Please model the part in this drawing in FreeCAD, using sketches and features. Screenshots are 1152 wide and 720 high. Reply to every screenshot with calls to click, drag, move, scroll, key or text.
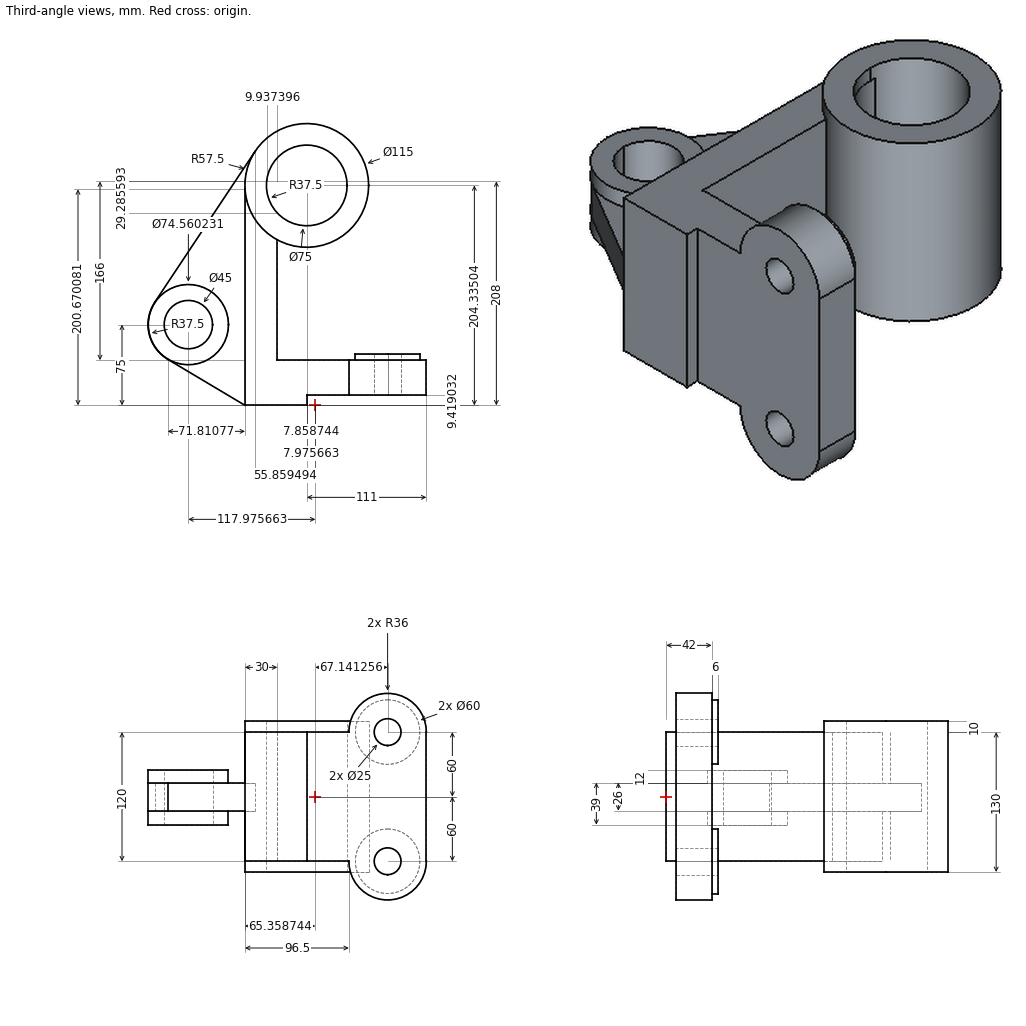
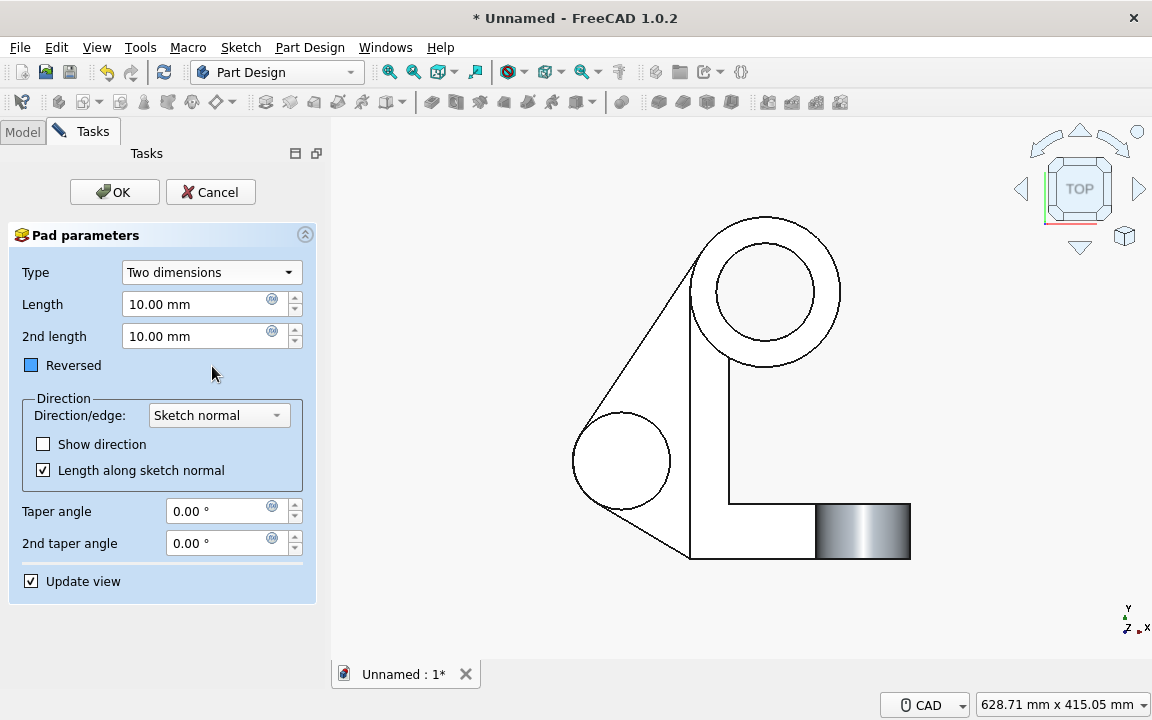
triple_click(204, 304)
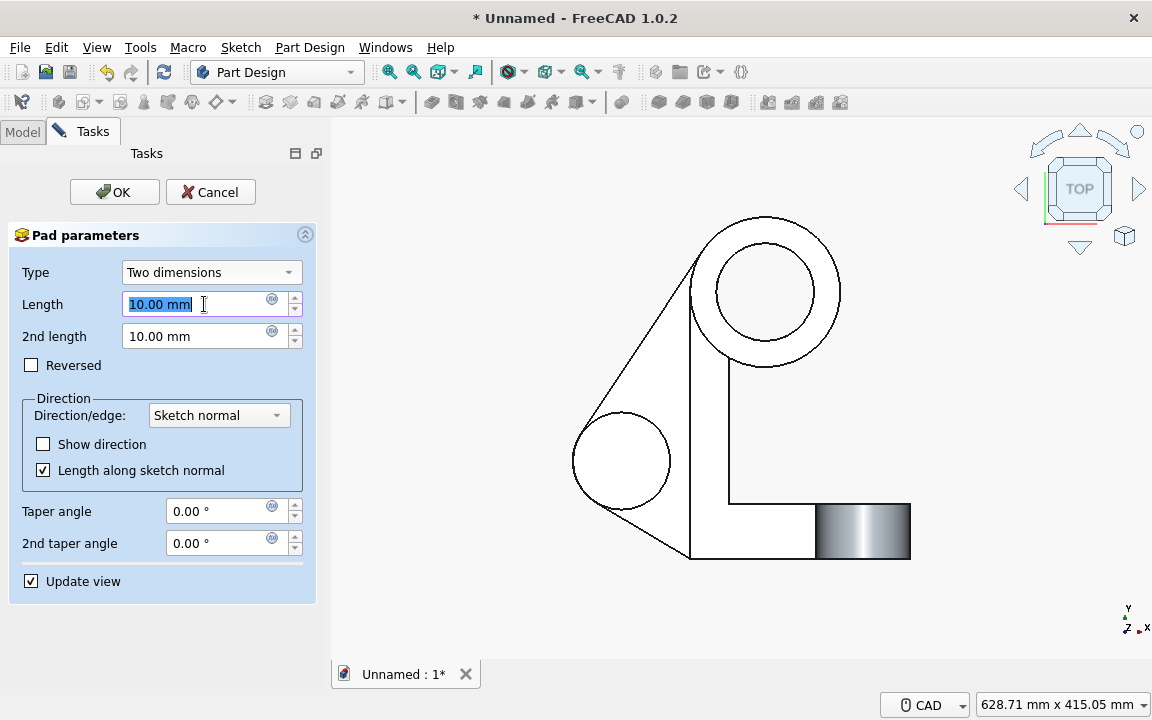
text(12)
key(Tab)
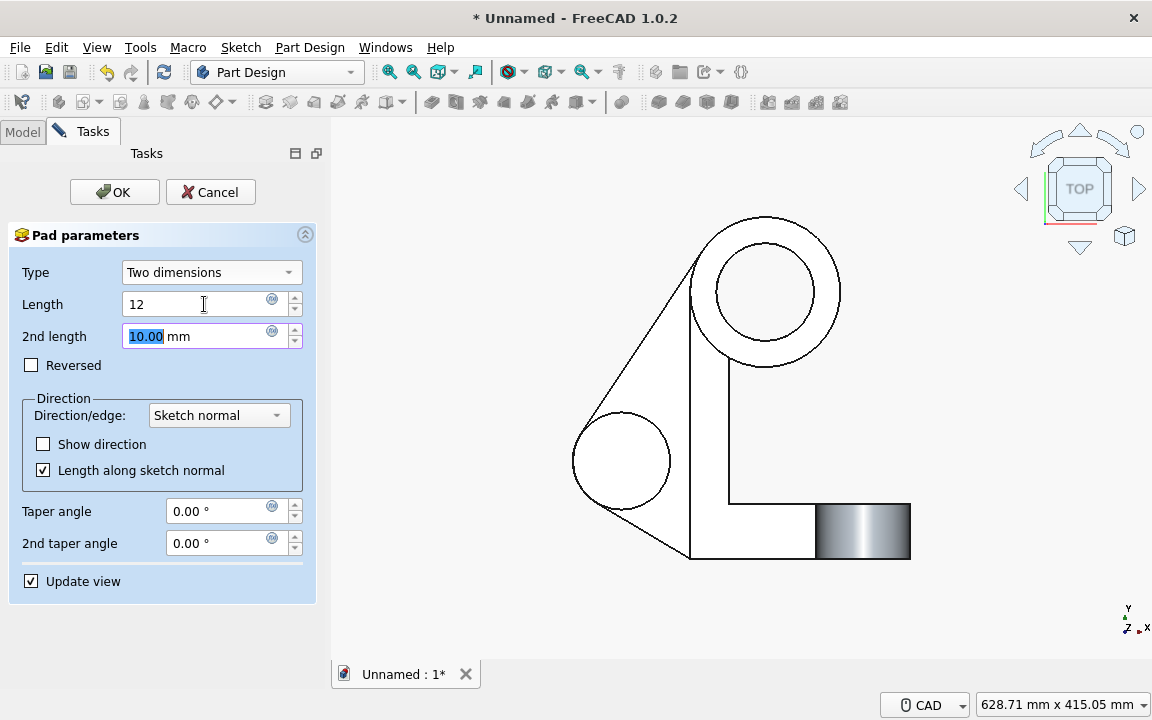
text(39)
key(Tab)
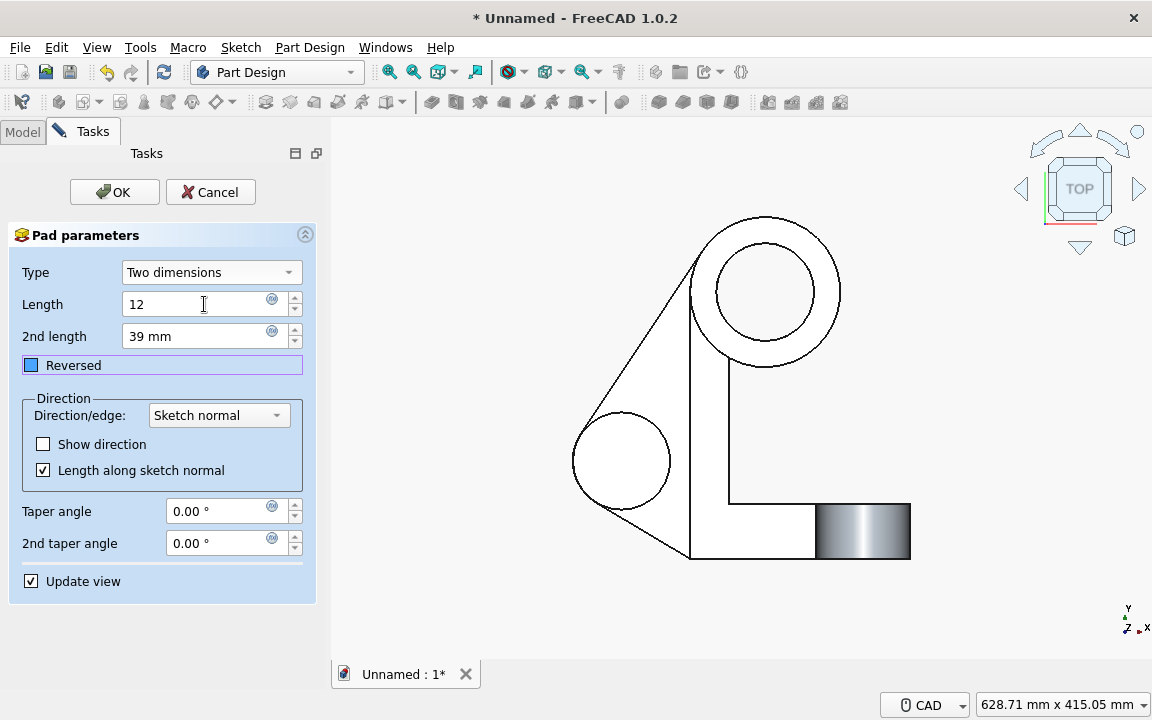
click(115, 192)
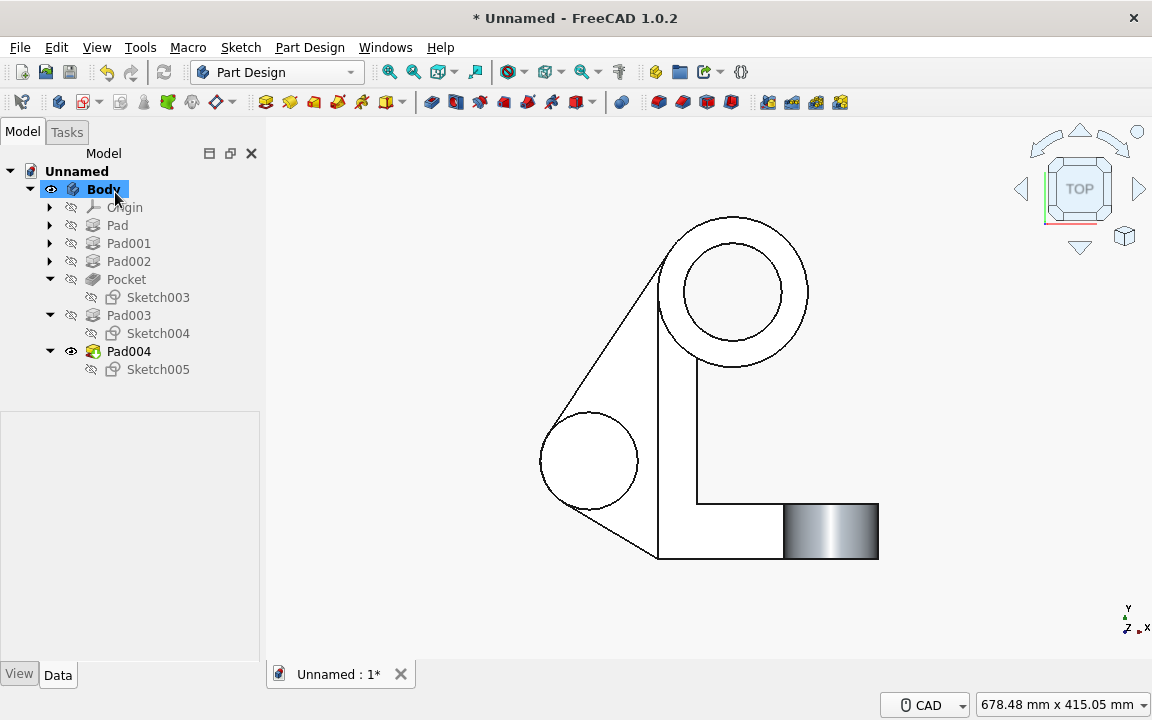
click(589, 460)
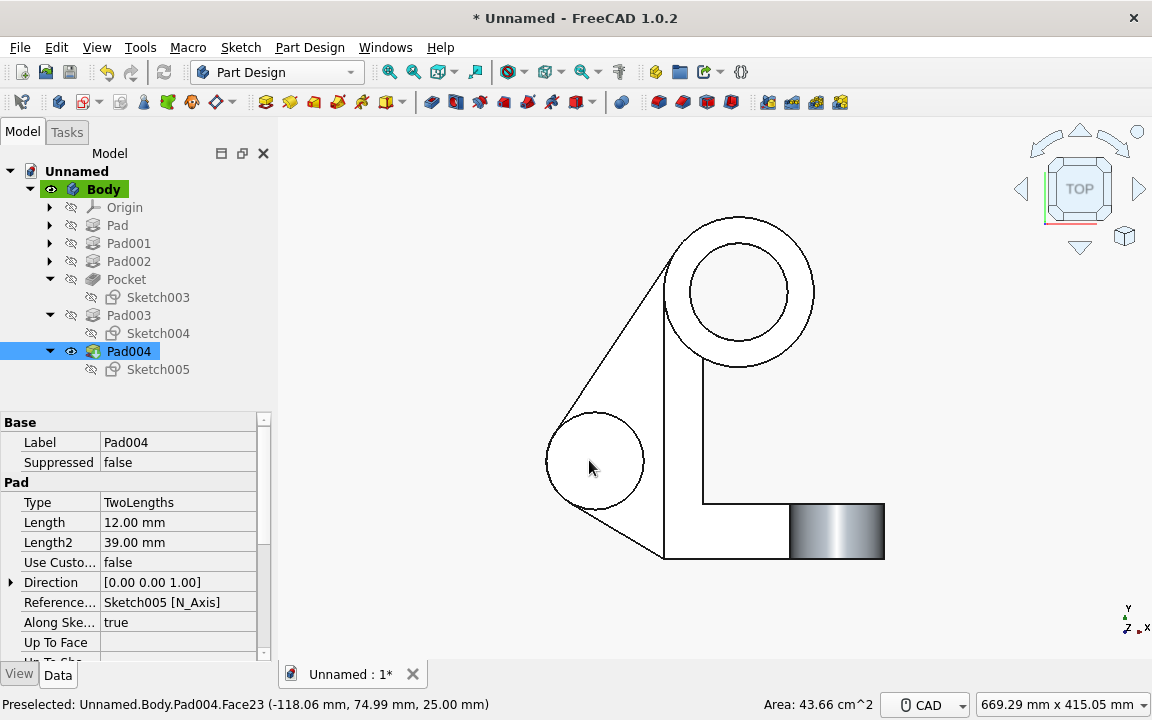
click(84, 102)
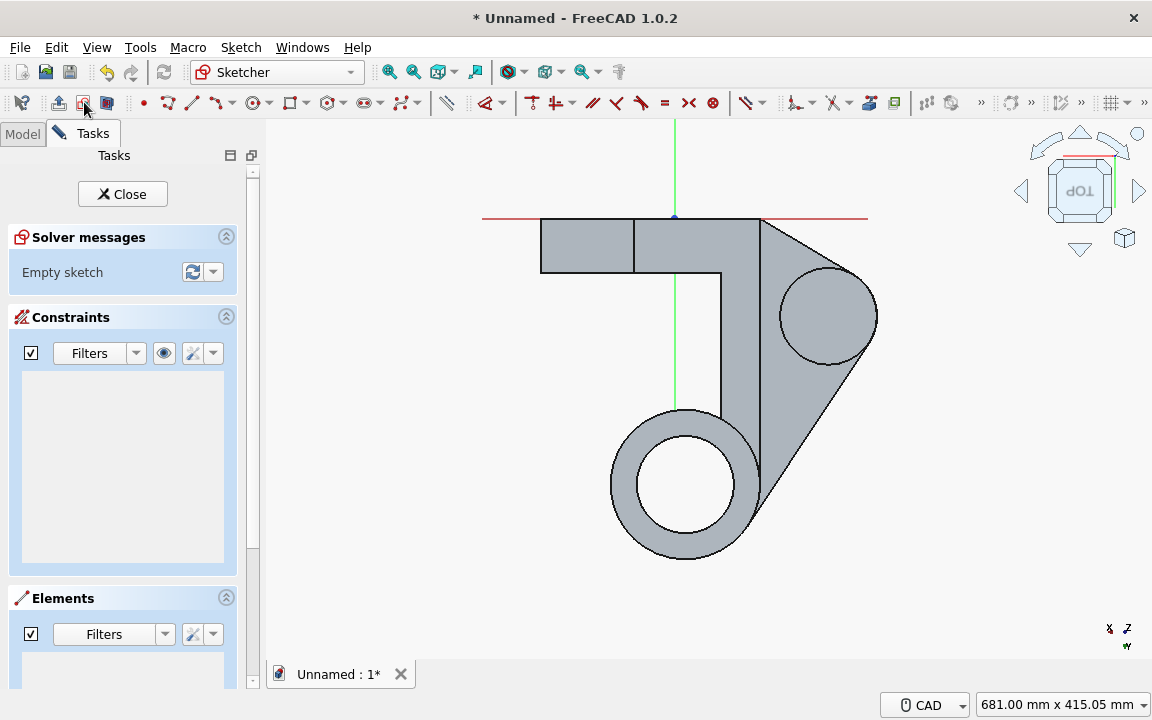
click(108, 104)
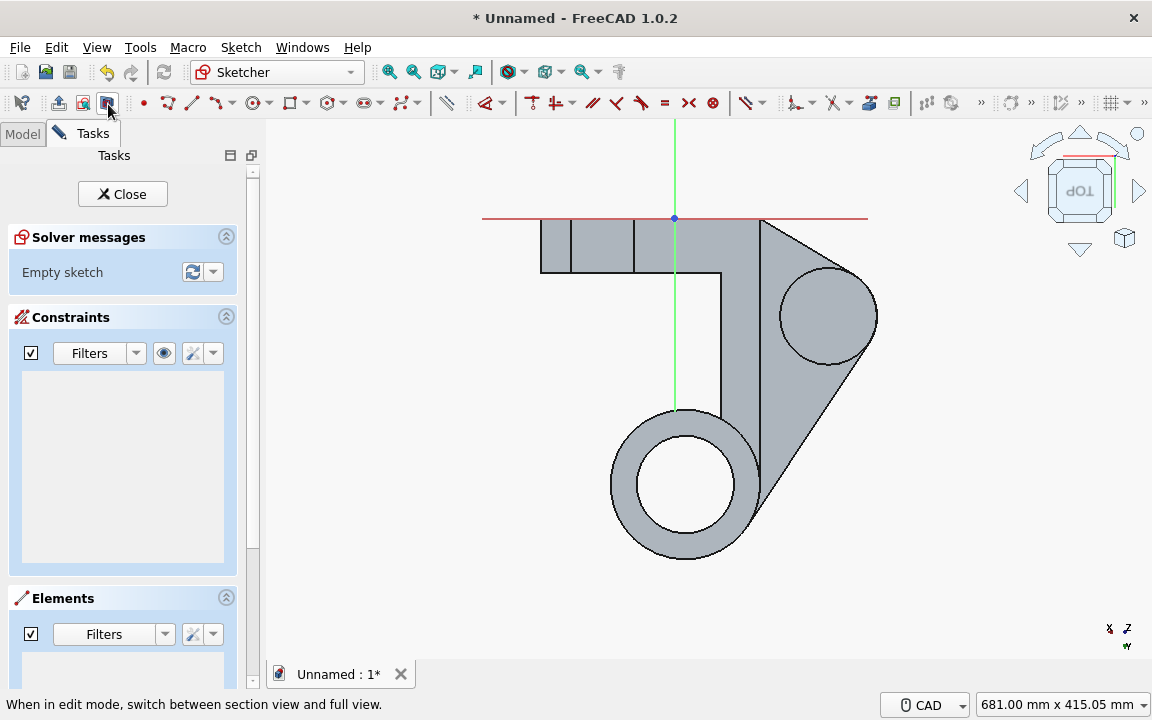
scroll(866, 302, up, 9)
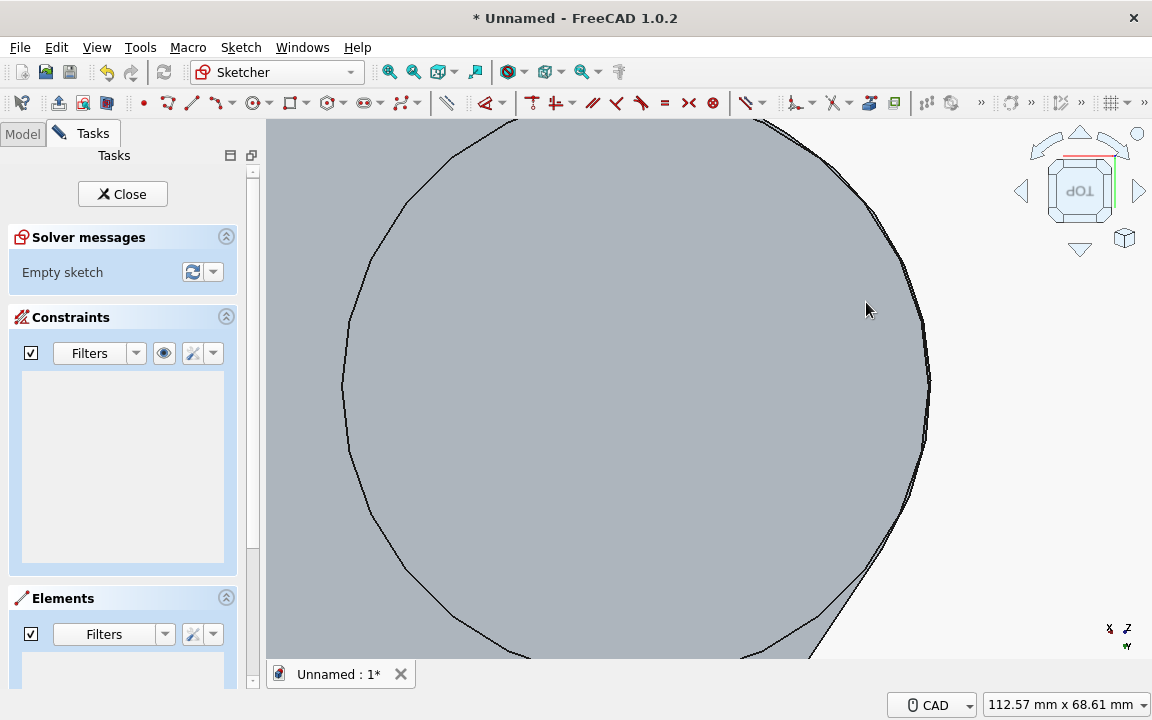
click(254, 104)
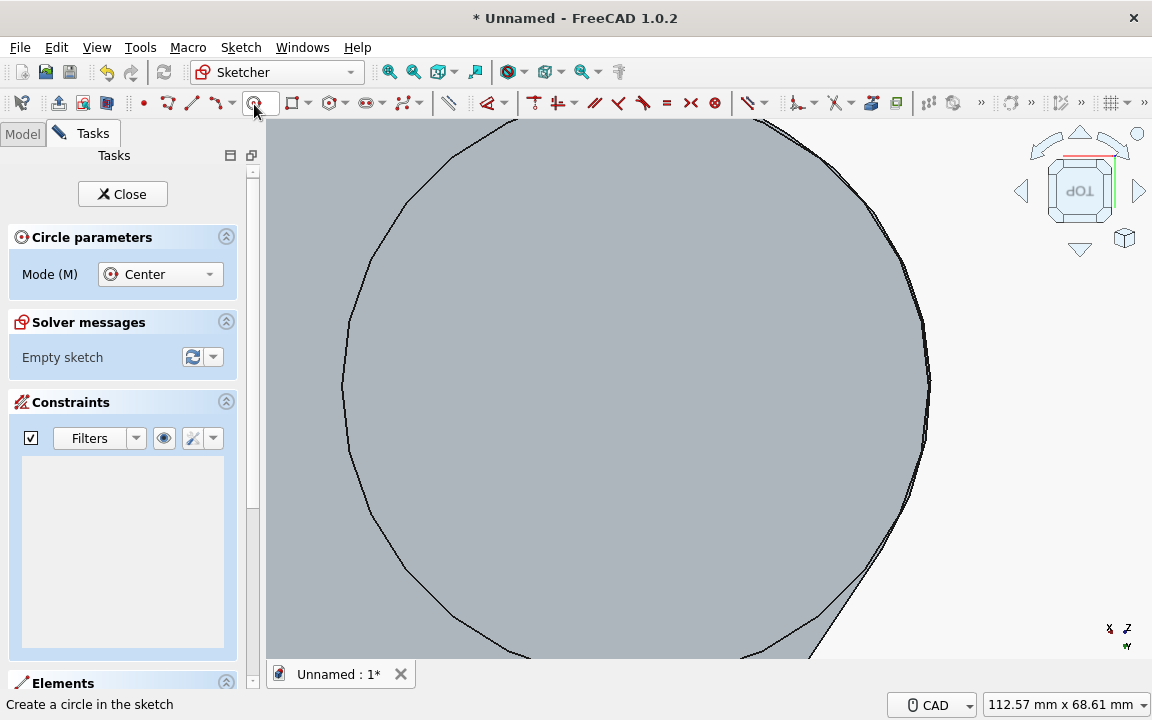
click(635, 387)
move(761, 261)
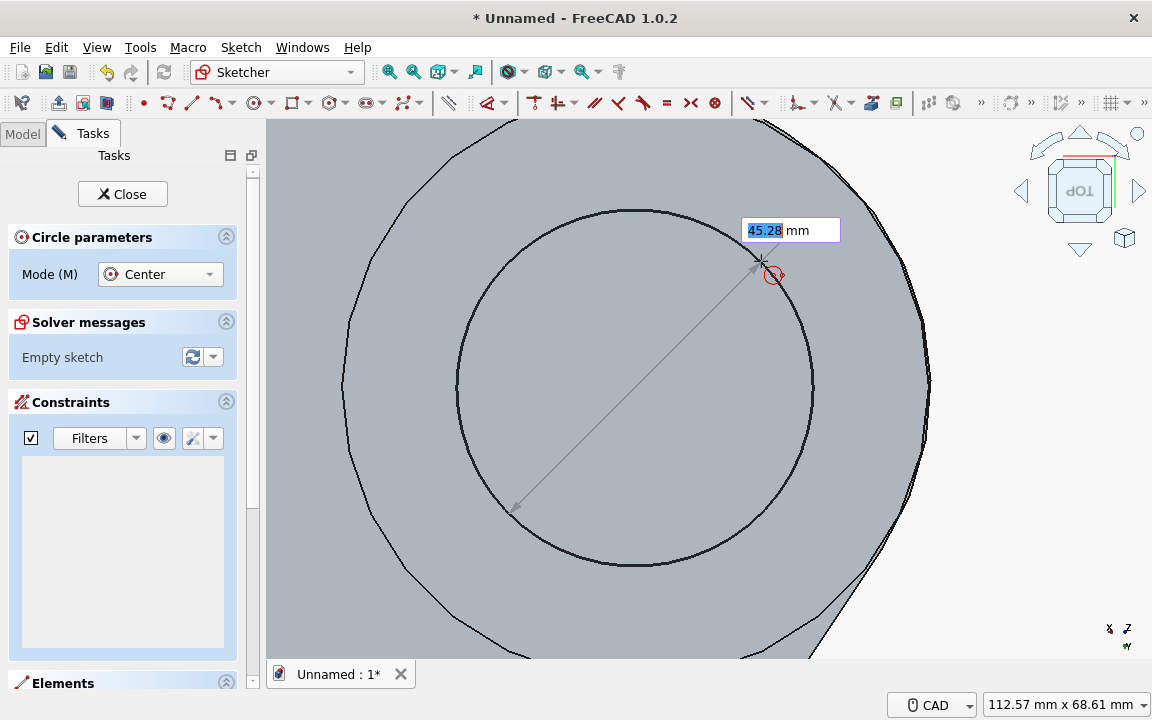
text(45)
key(Return)
key(Escape)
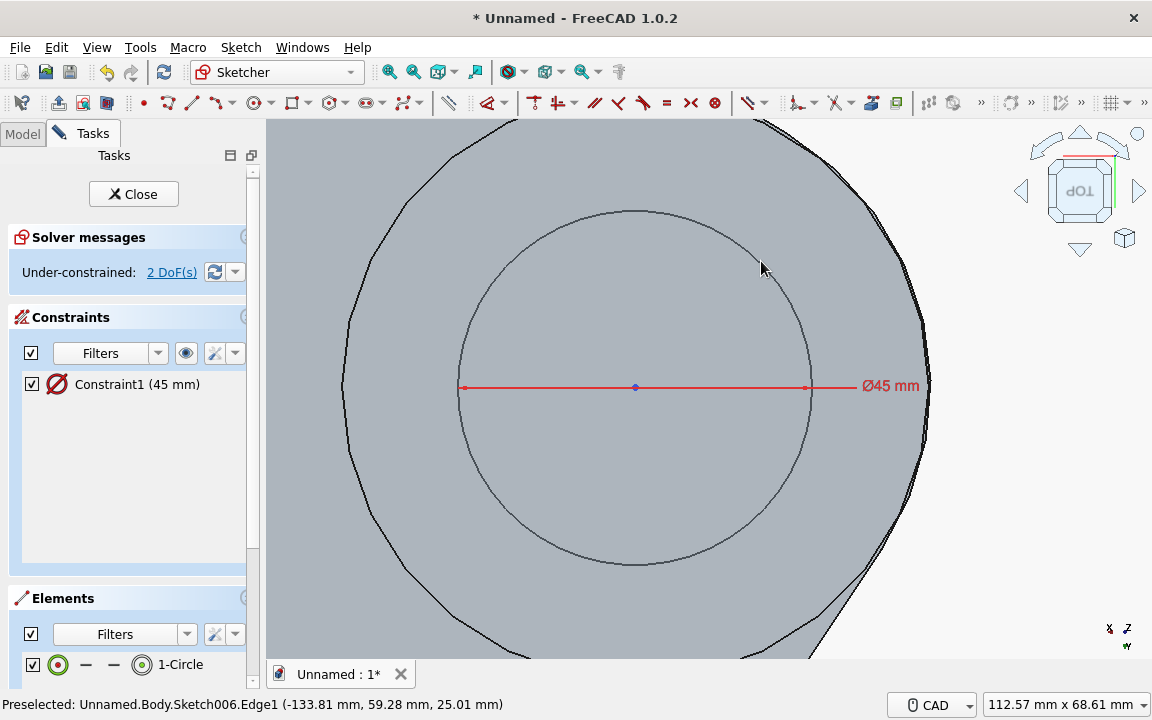
click(488, 104)